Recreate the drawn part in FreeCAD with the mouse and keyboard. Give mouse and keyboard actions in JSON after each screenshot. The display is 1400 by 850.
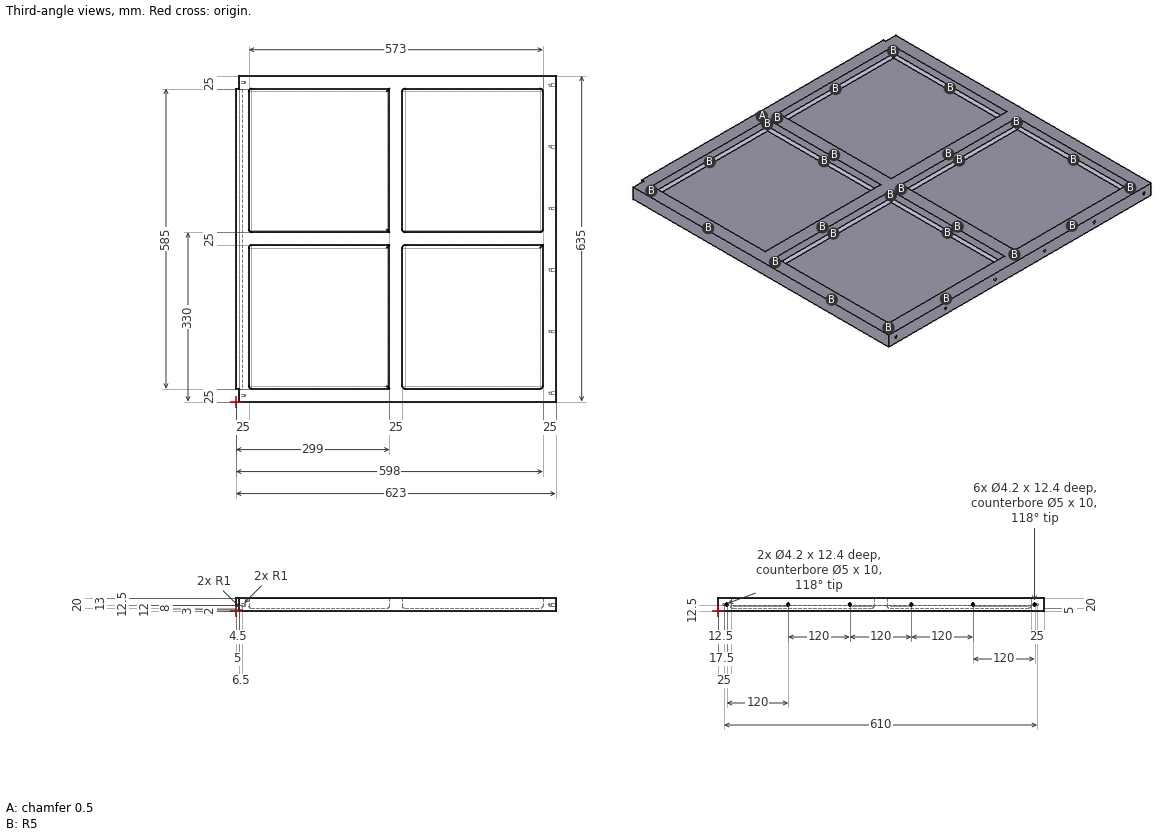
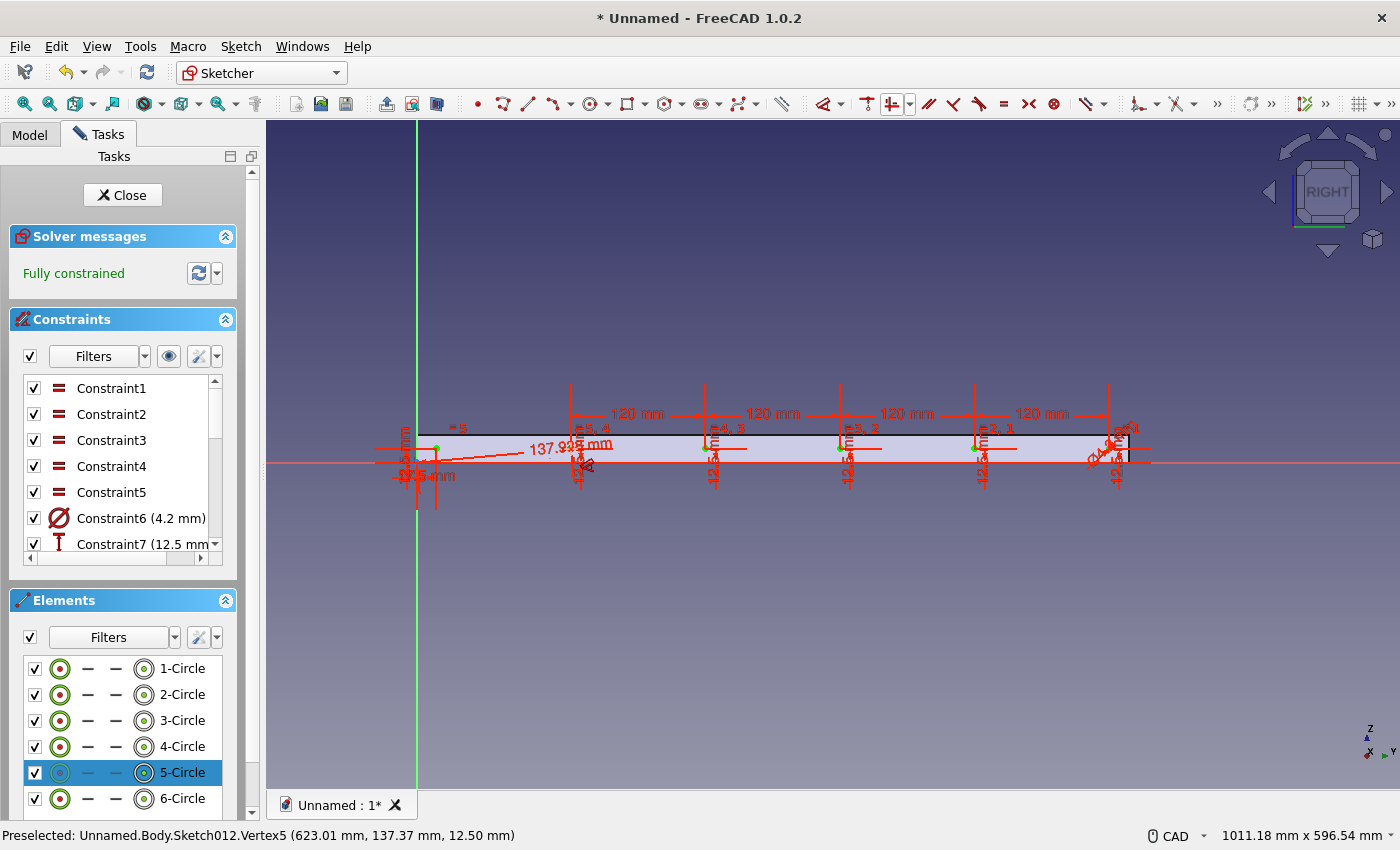
{"action": "left_click", "coordinate": [436, 449]}
{"action": "left_click", "coordinate": [504, 415]}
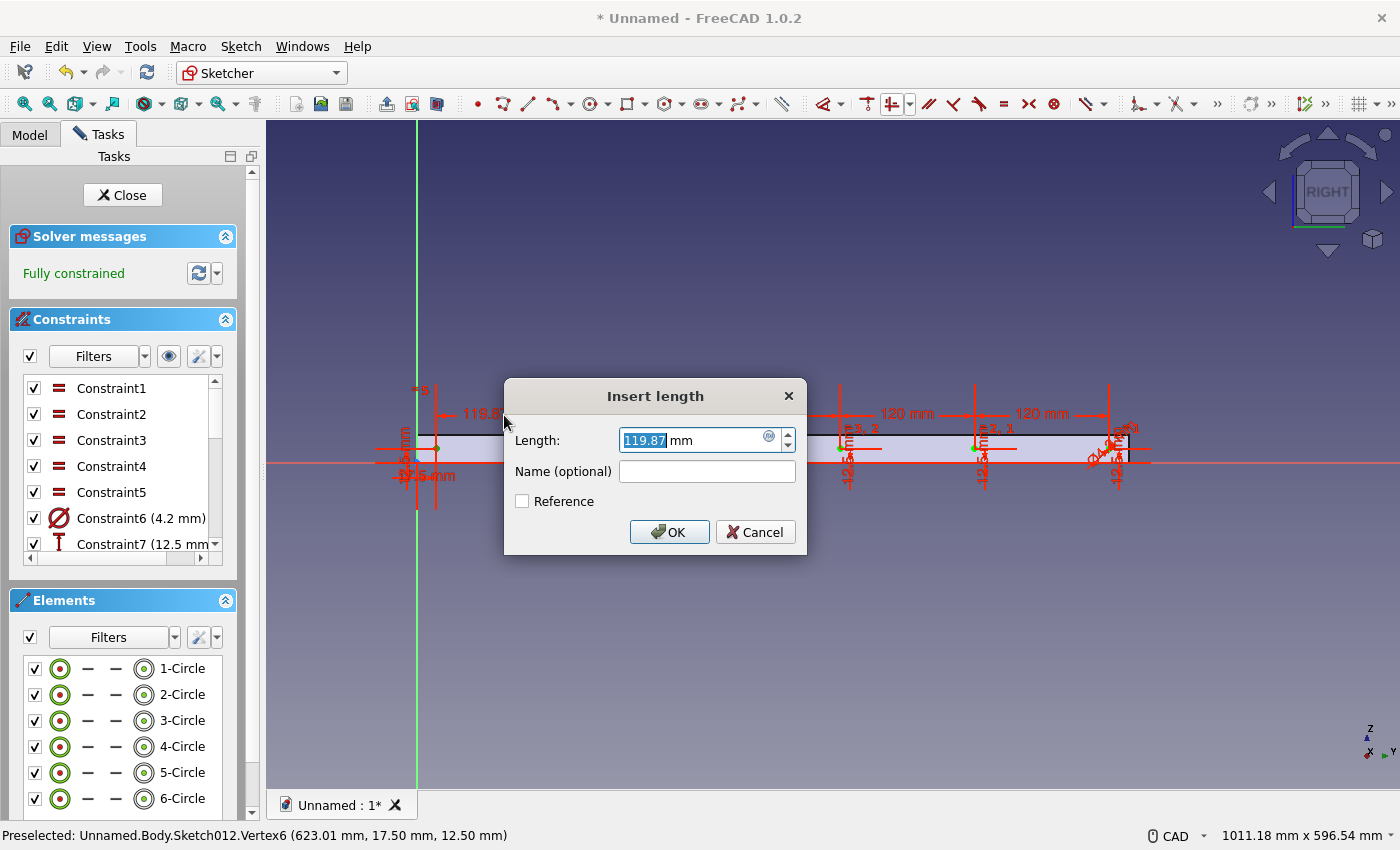
{"action": "type", "text": "120"}
{"action": "key", "text": "Return"}
{"action": "key", "text": "Escape"}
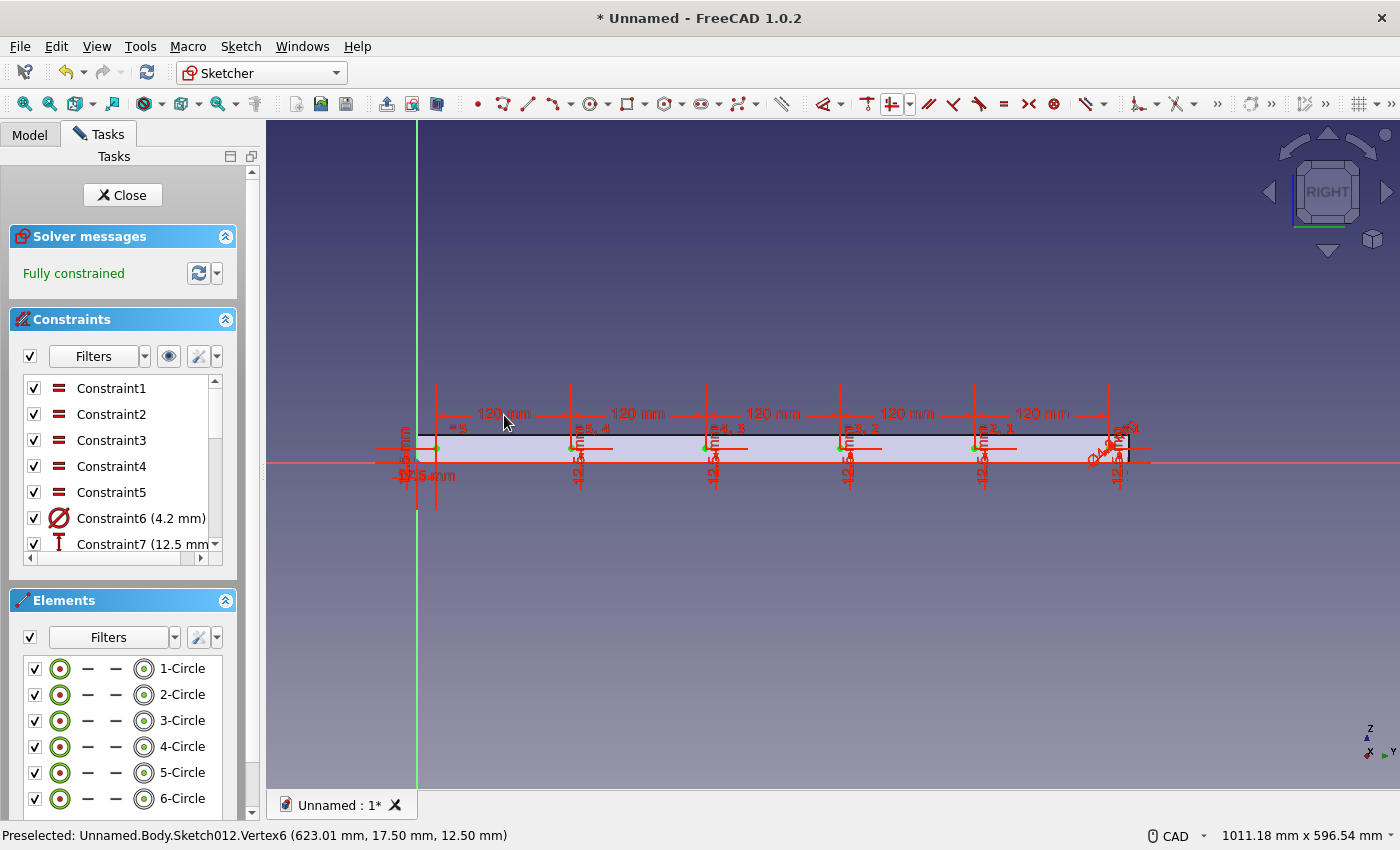
{"action": "left_click", "coordinate": [123, 195]}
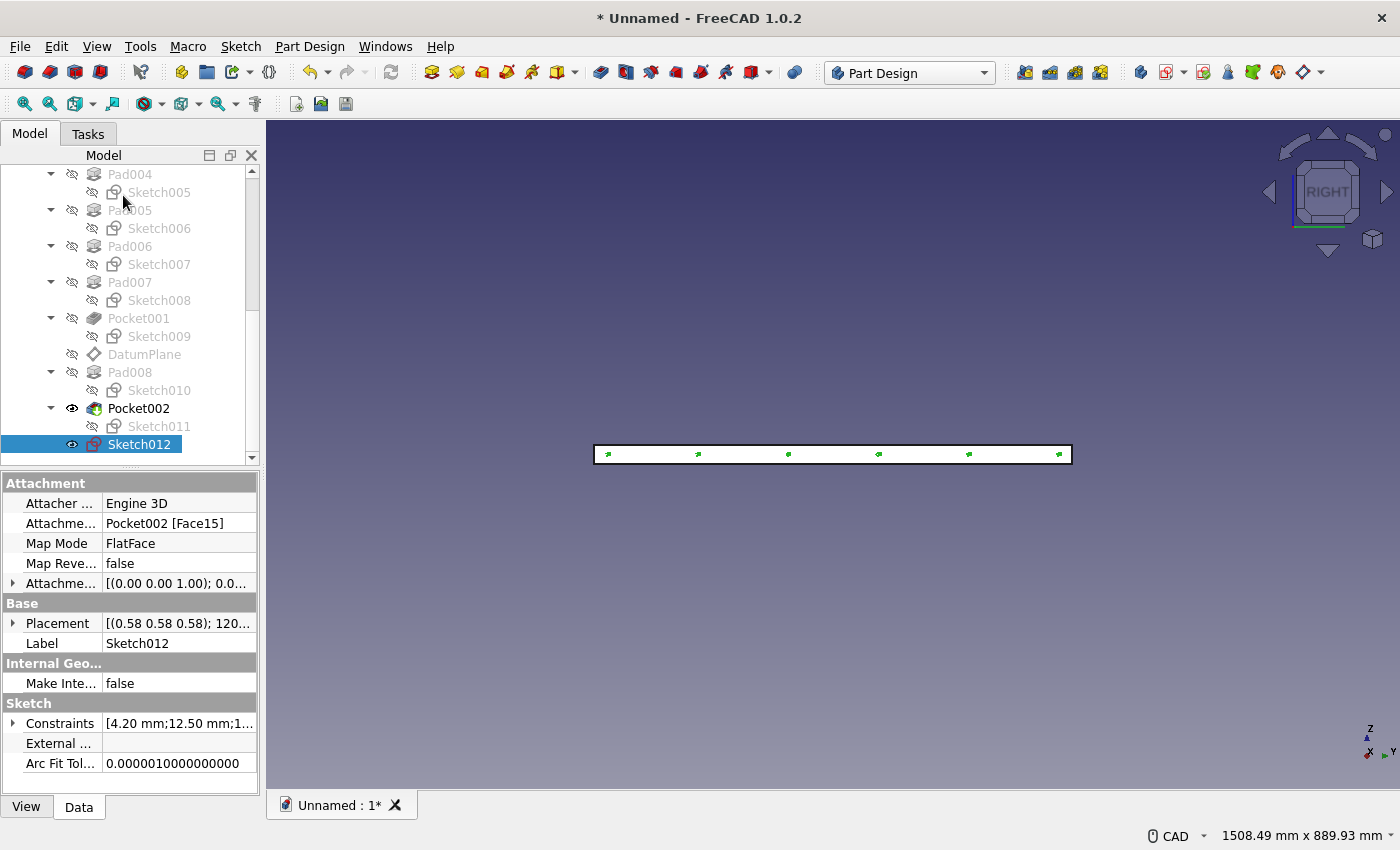
{"action": "left_click", "coordinate": [626, 72]}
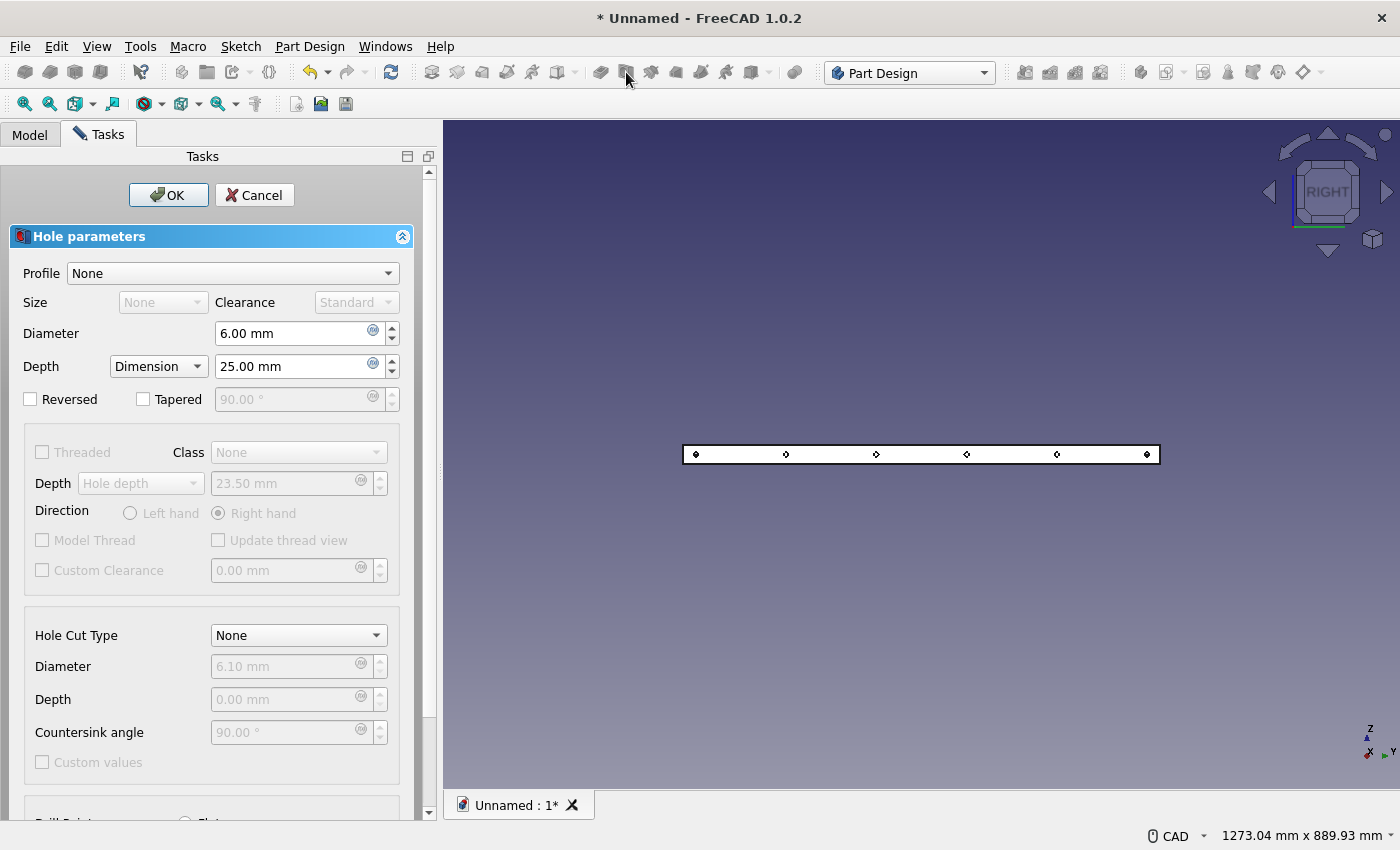
{"action": "triple_click", "coordinate": [300, 334]}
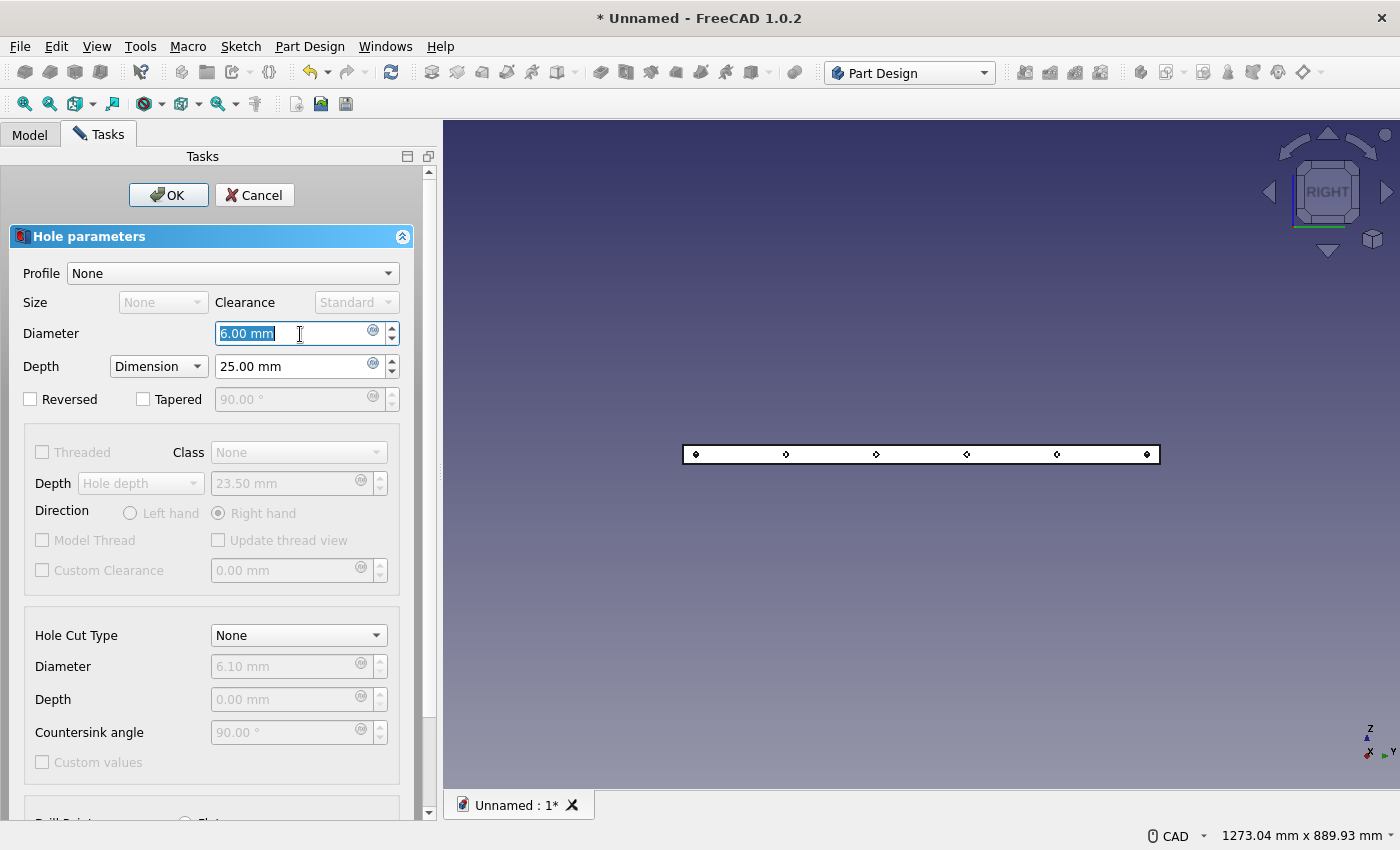
{"action": "type", "text": "4.2"}
{"action": "key", "text": "Tab"}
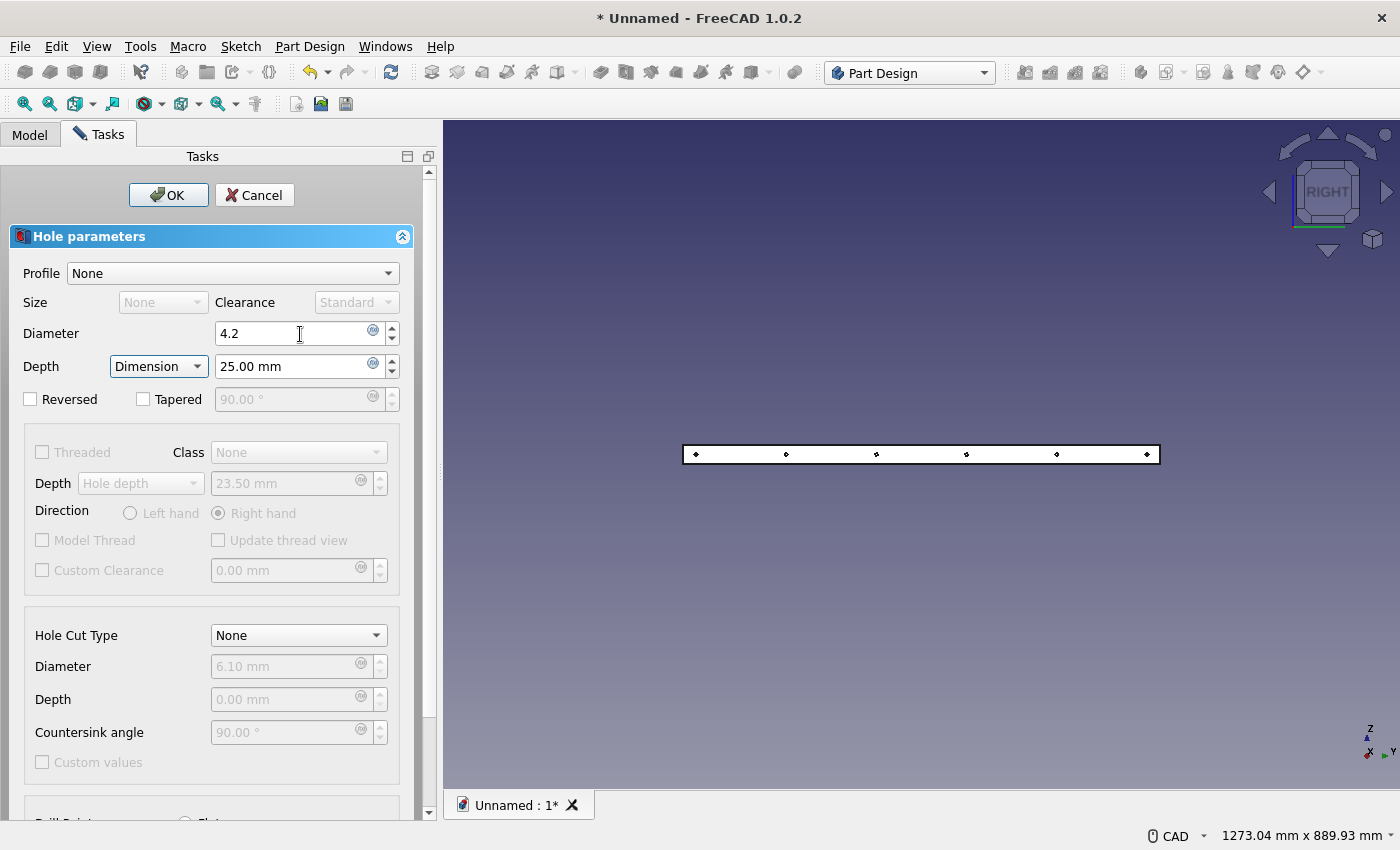
{"action": "triple_click", "coordinate": [300, 366]}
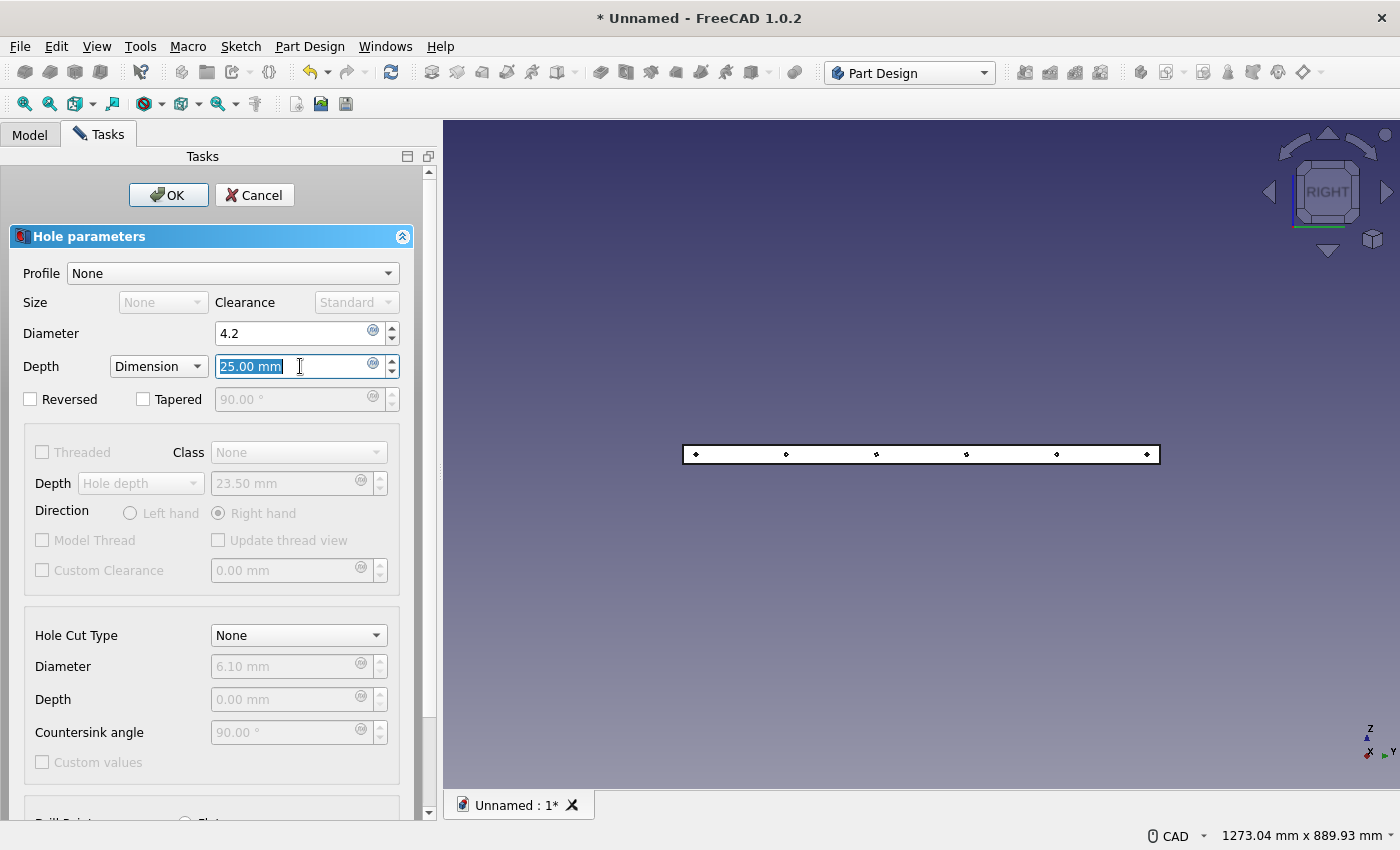
{"action": "type", "text": "12.4"}
{"action": "key", "text": "Tab"}